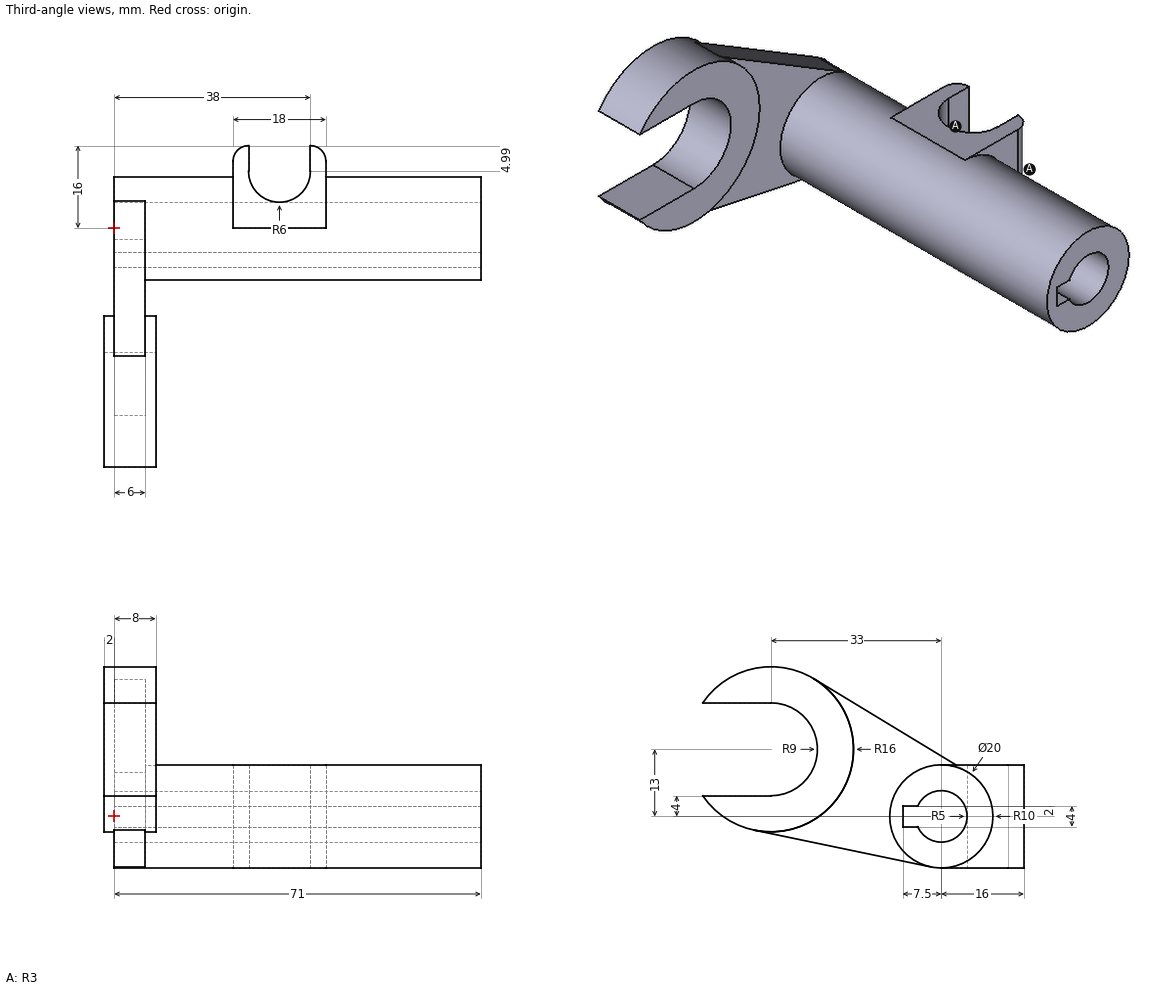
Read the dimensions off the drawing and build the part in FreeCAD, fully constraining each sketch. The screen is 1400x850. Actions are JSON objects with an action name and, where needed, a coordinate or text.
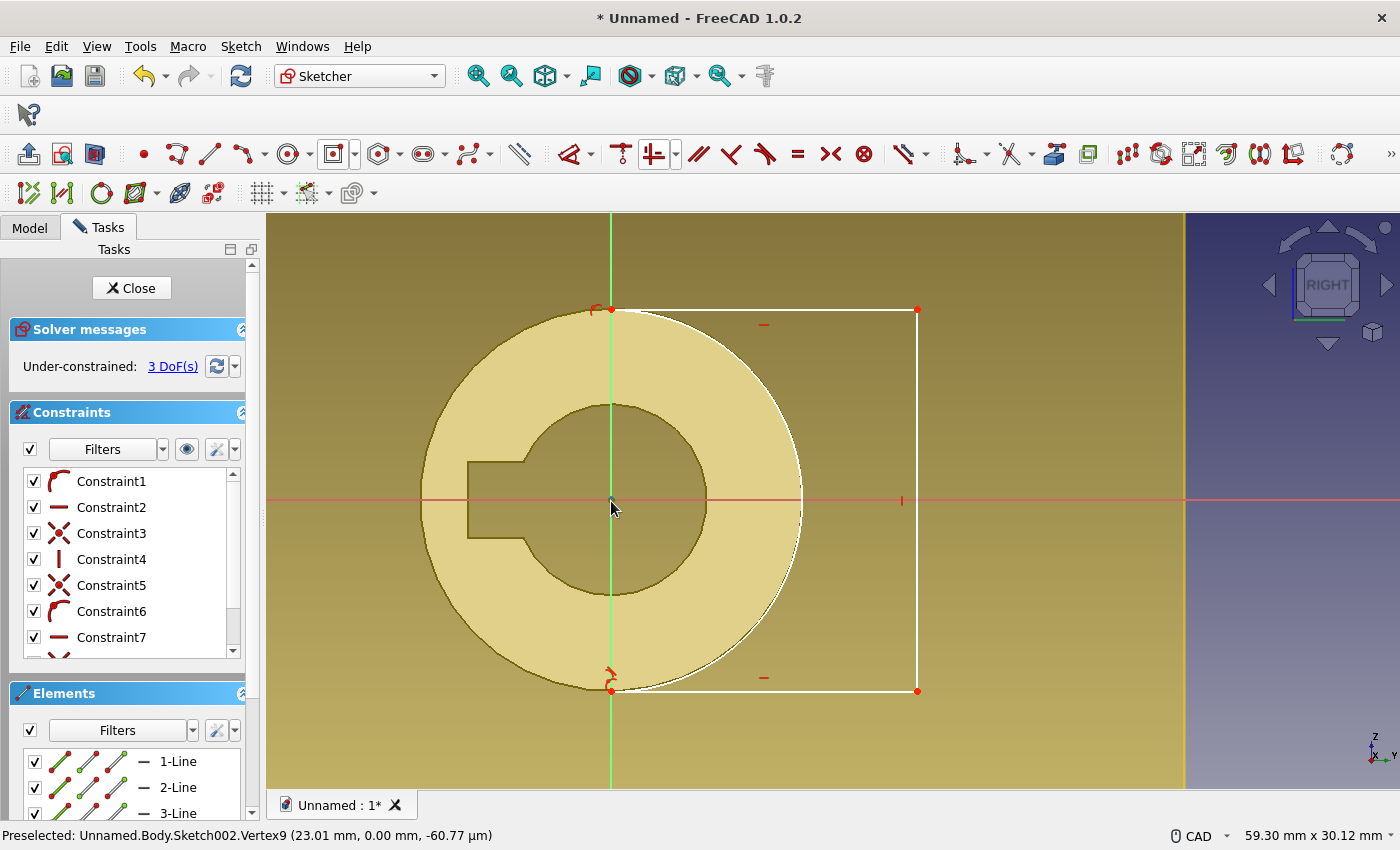
{"action": "left_click", "coordinate": [361, 500]}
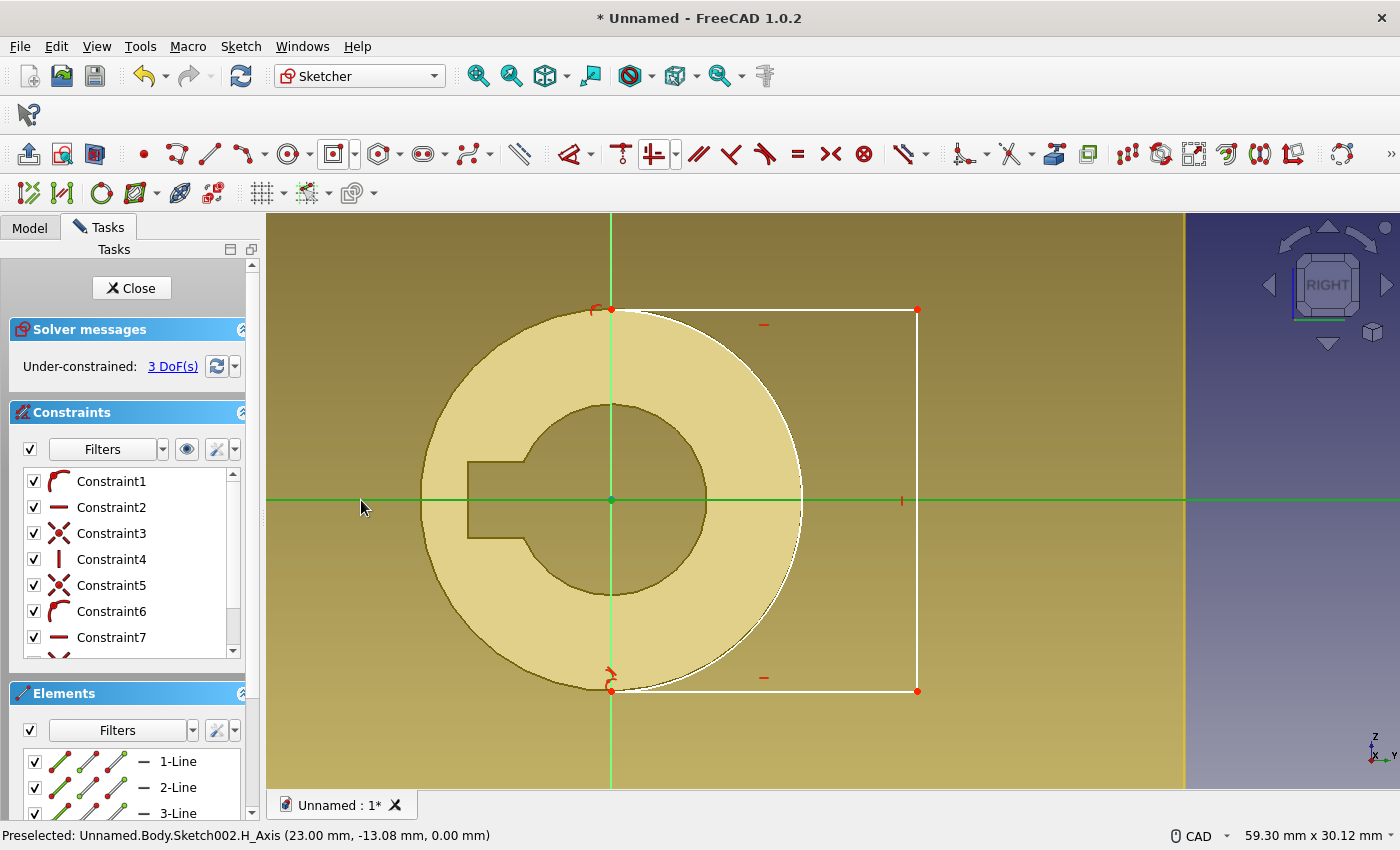
{"action": "key", "text": "c"}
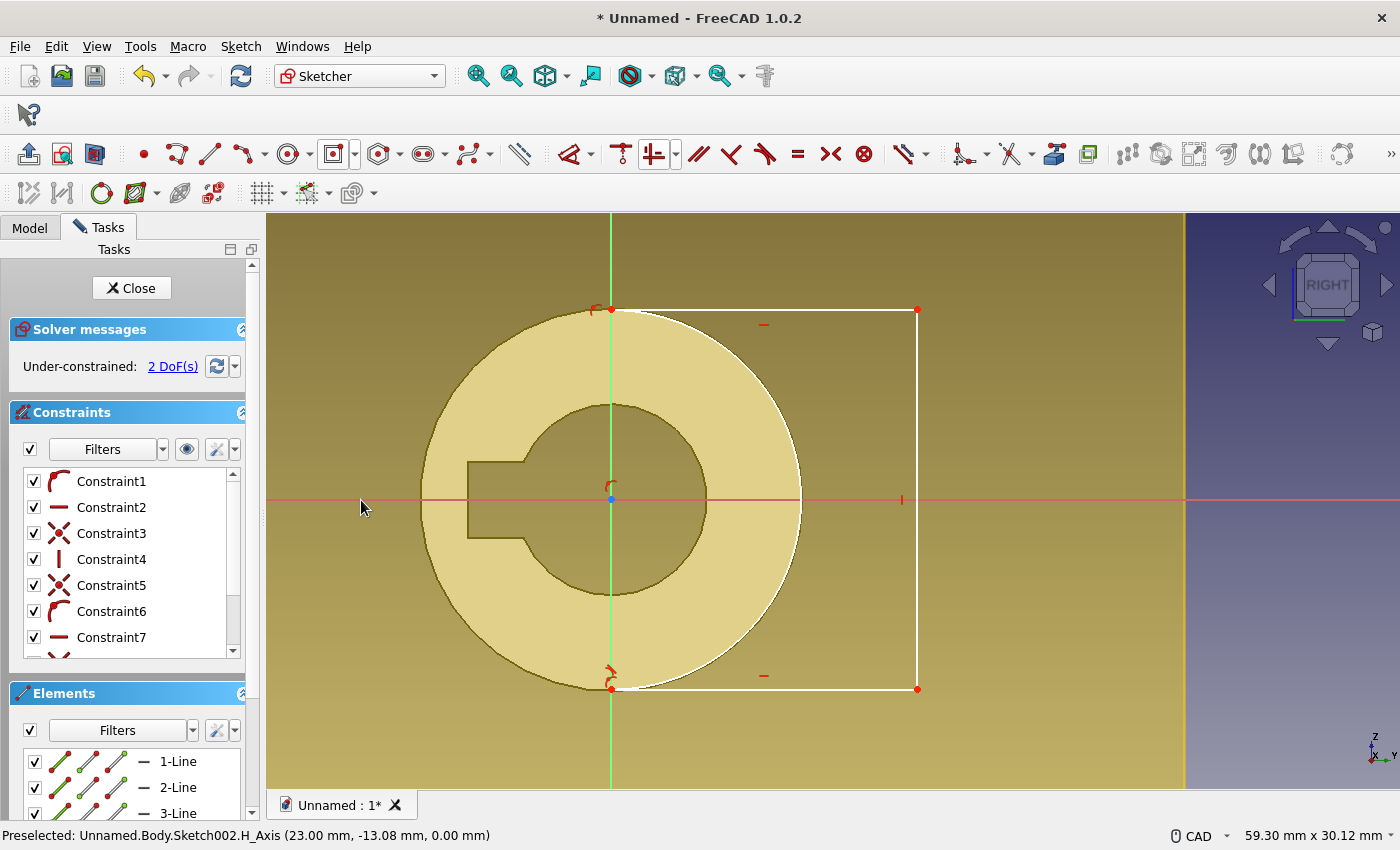
{"action": "key", "text": "d"}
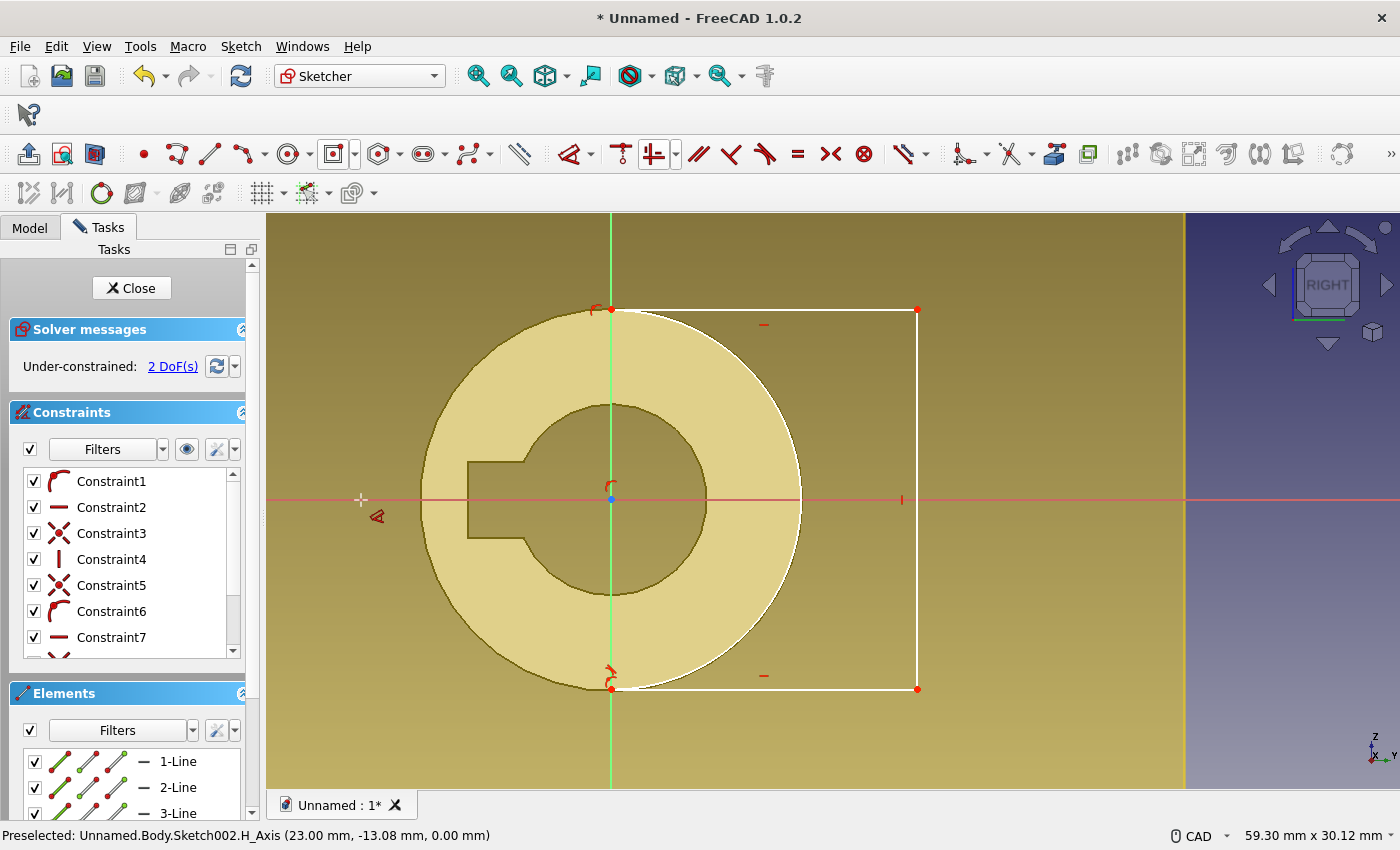
{"action": "left_click", "coordinate": [765, 611]}
{"action": "left_click", "coordinate": [791, 630]}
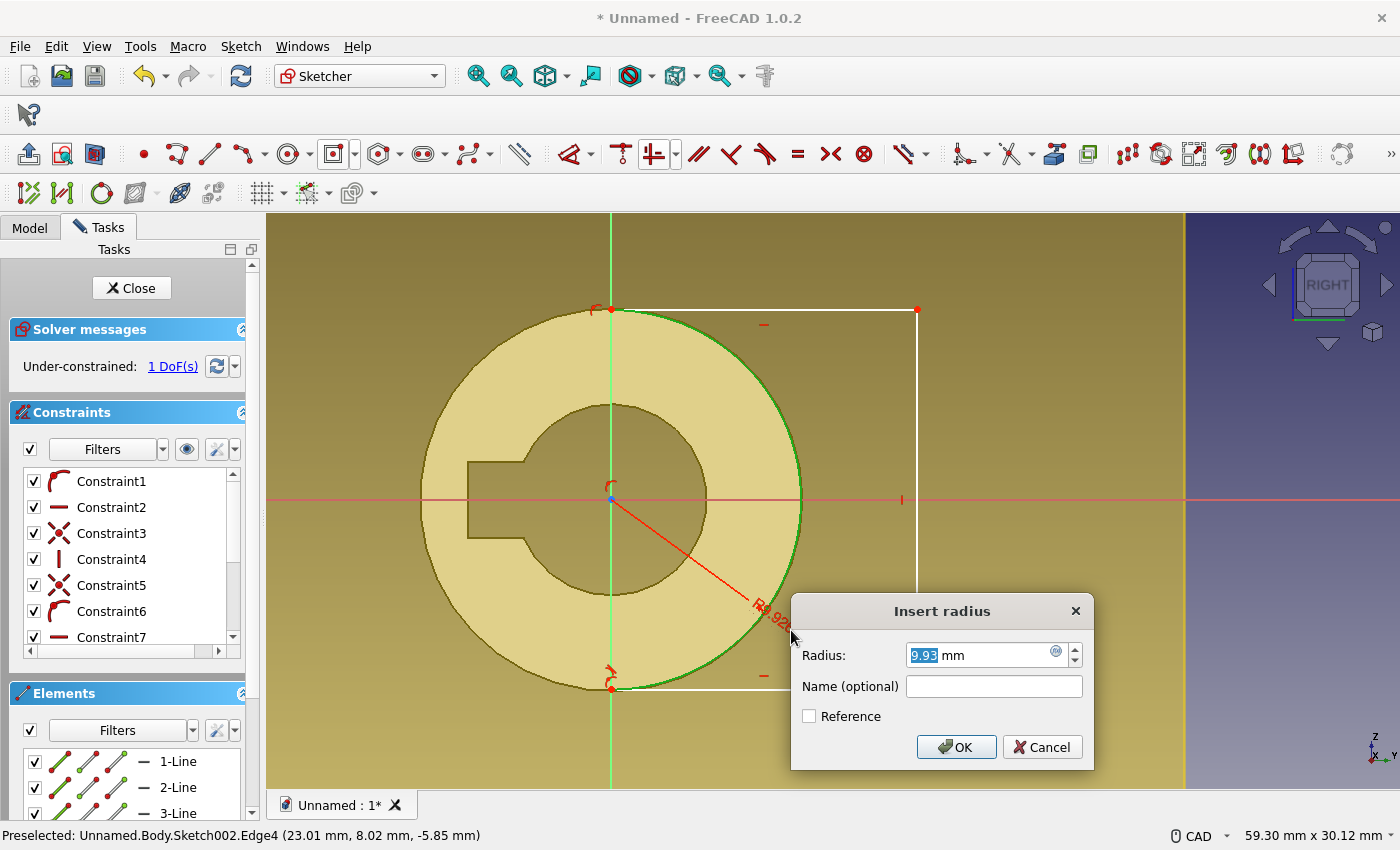
{"action": "type", "text": "10"}
{"action": "key", "text": "Return"}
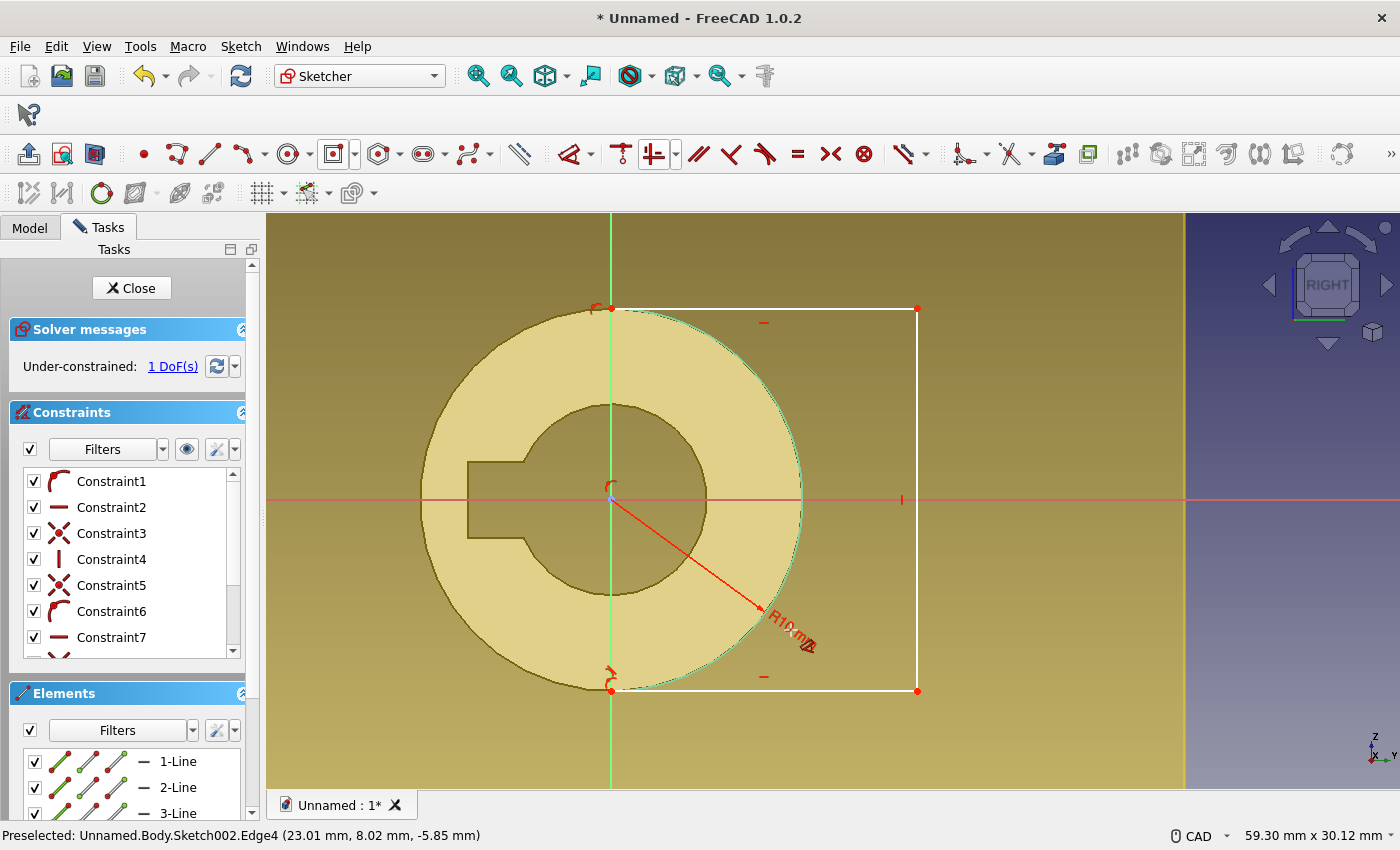
{"action": "left_click", "coordinate": [703, 691]}
{"action": "left_click", "coordinate": [764, 725]}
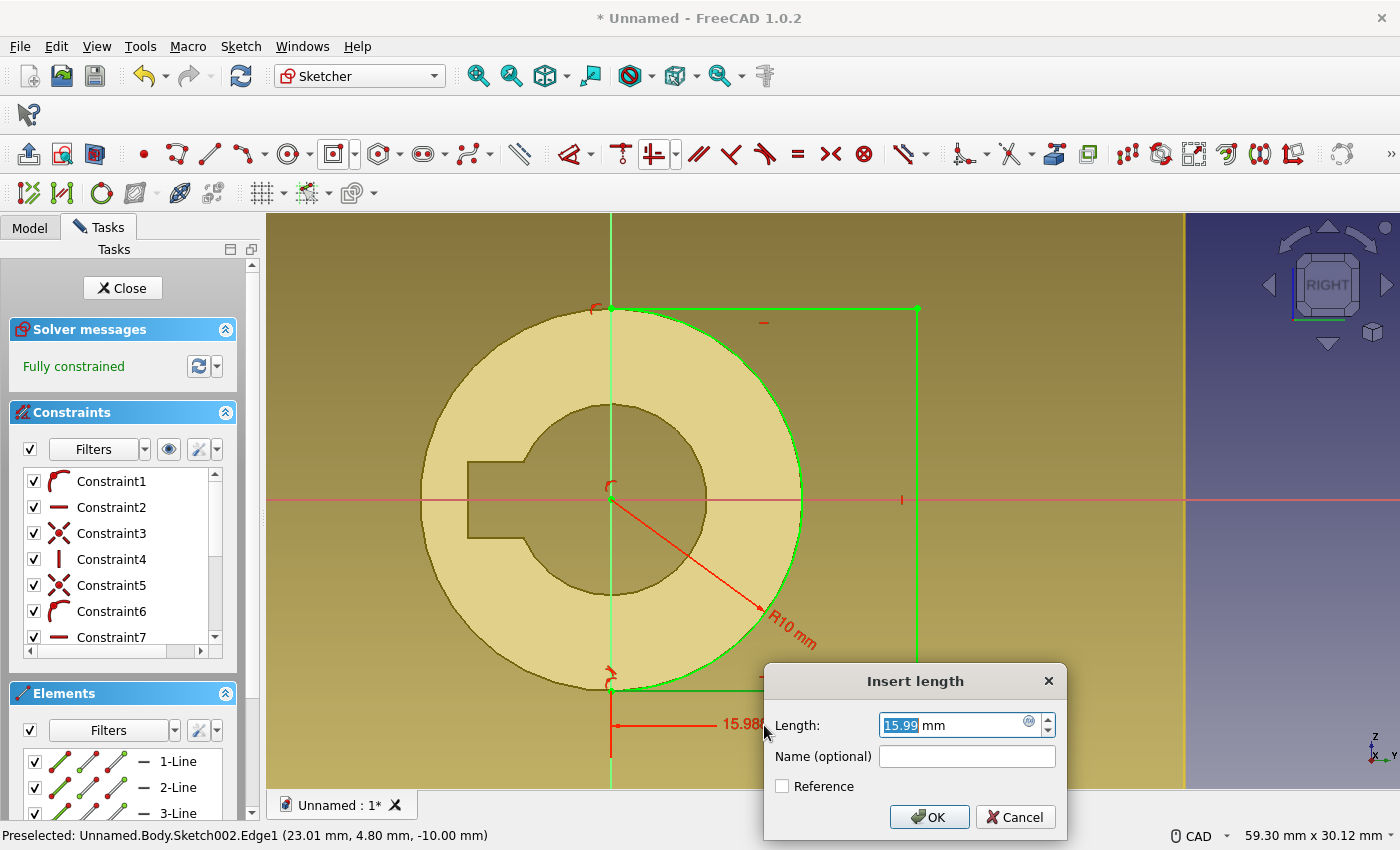
{"action": "type", "text": "16"}
{"action": "key", "text": "Return"}
{"action": "key", "text": "Escape"}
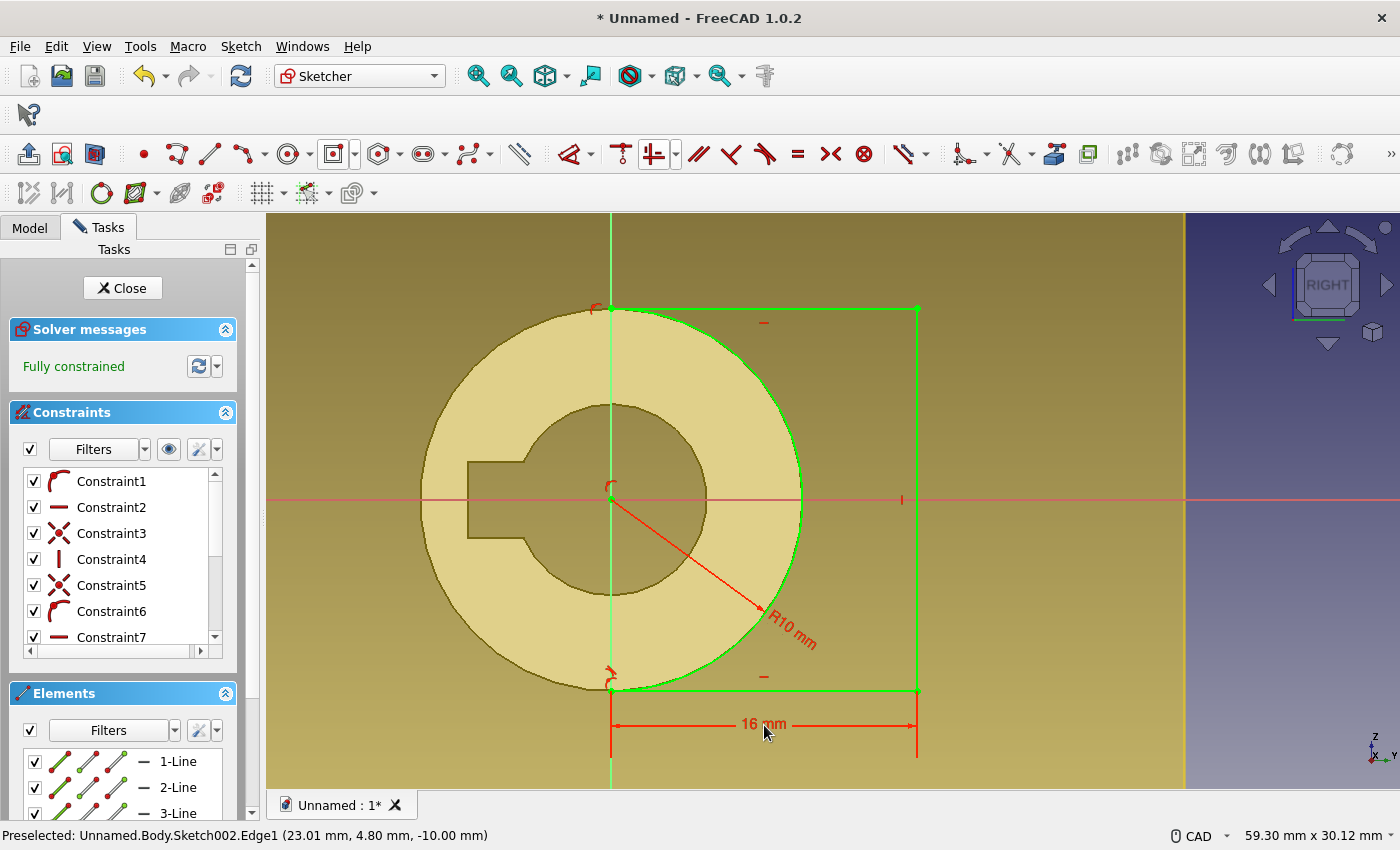
{"action": "left_click", "coordinate": [123, 288]}